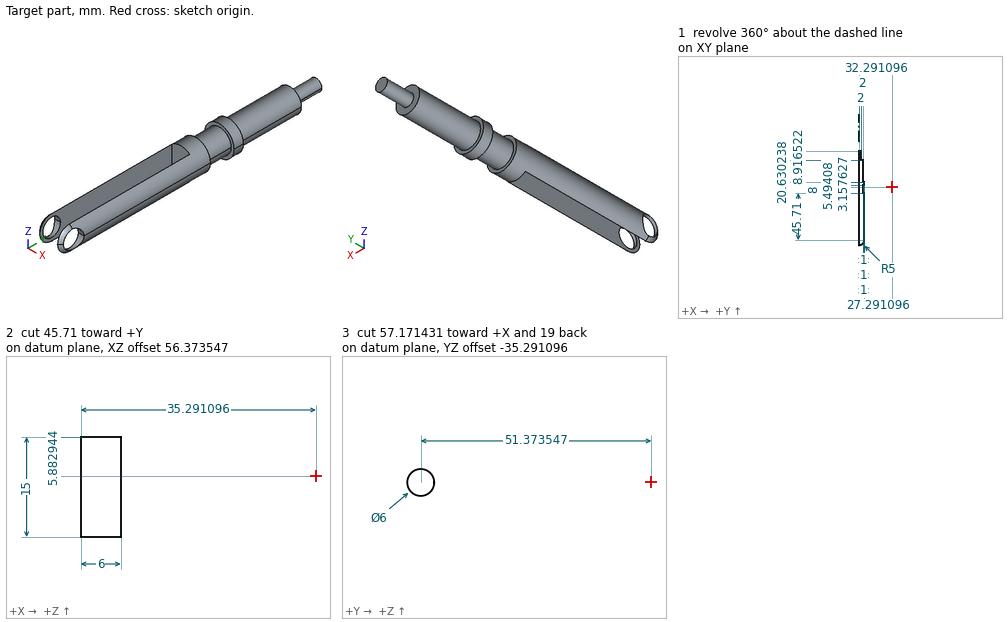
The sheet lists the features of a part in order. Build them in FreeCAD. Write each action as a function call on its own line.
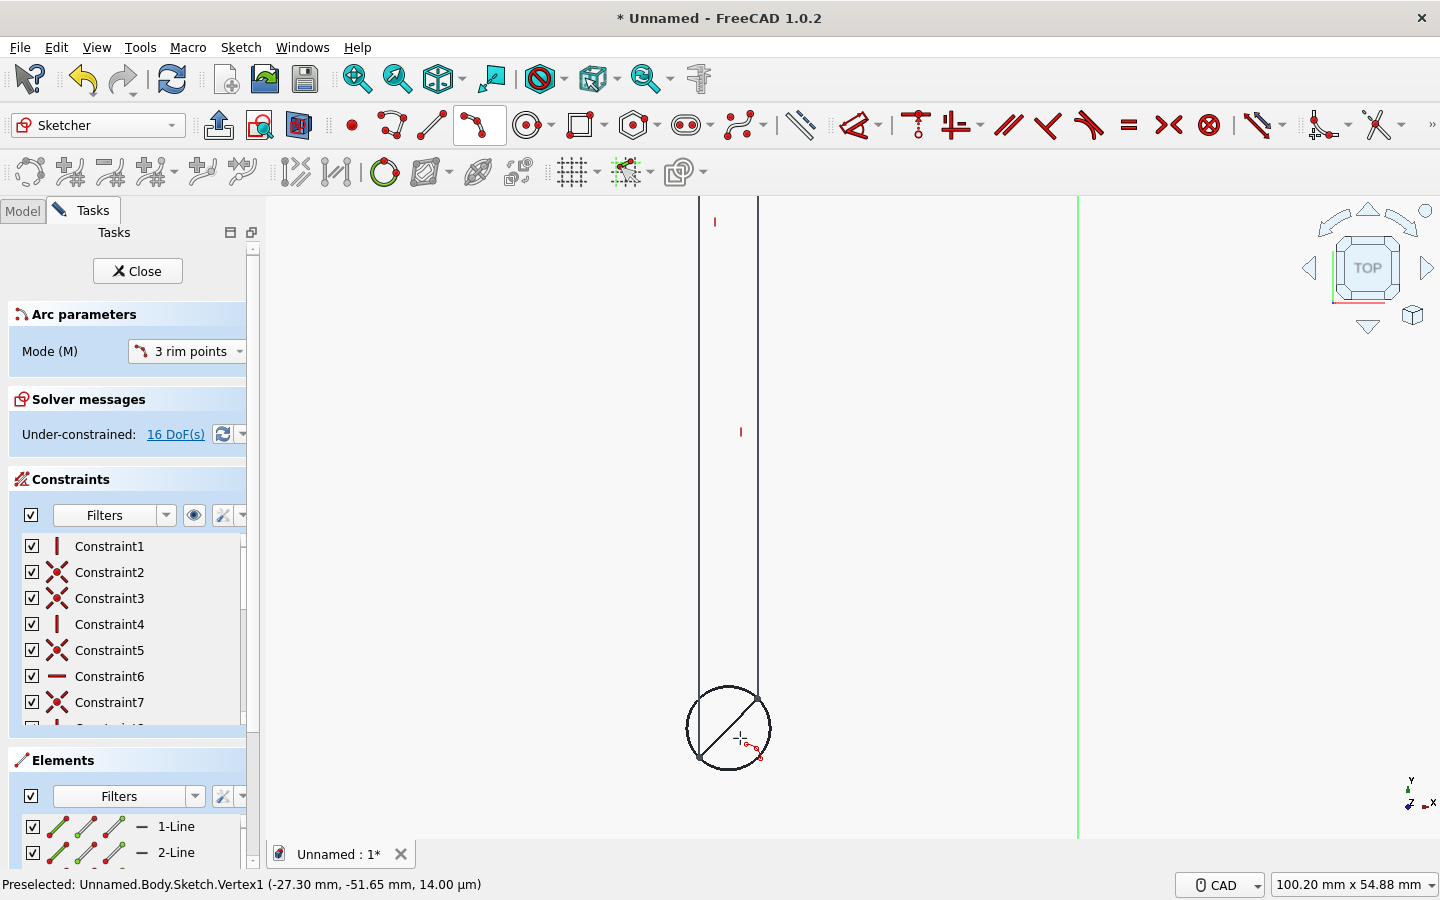
click(741, 737)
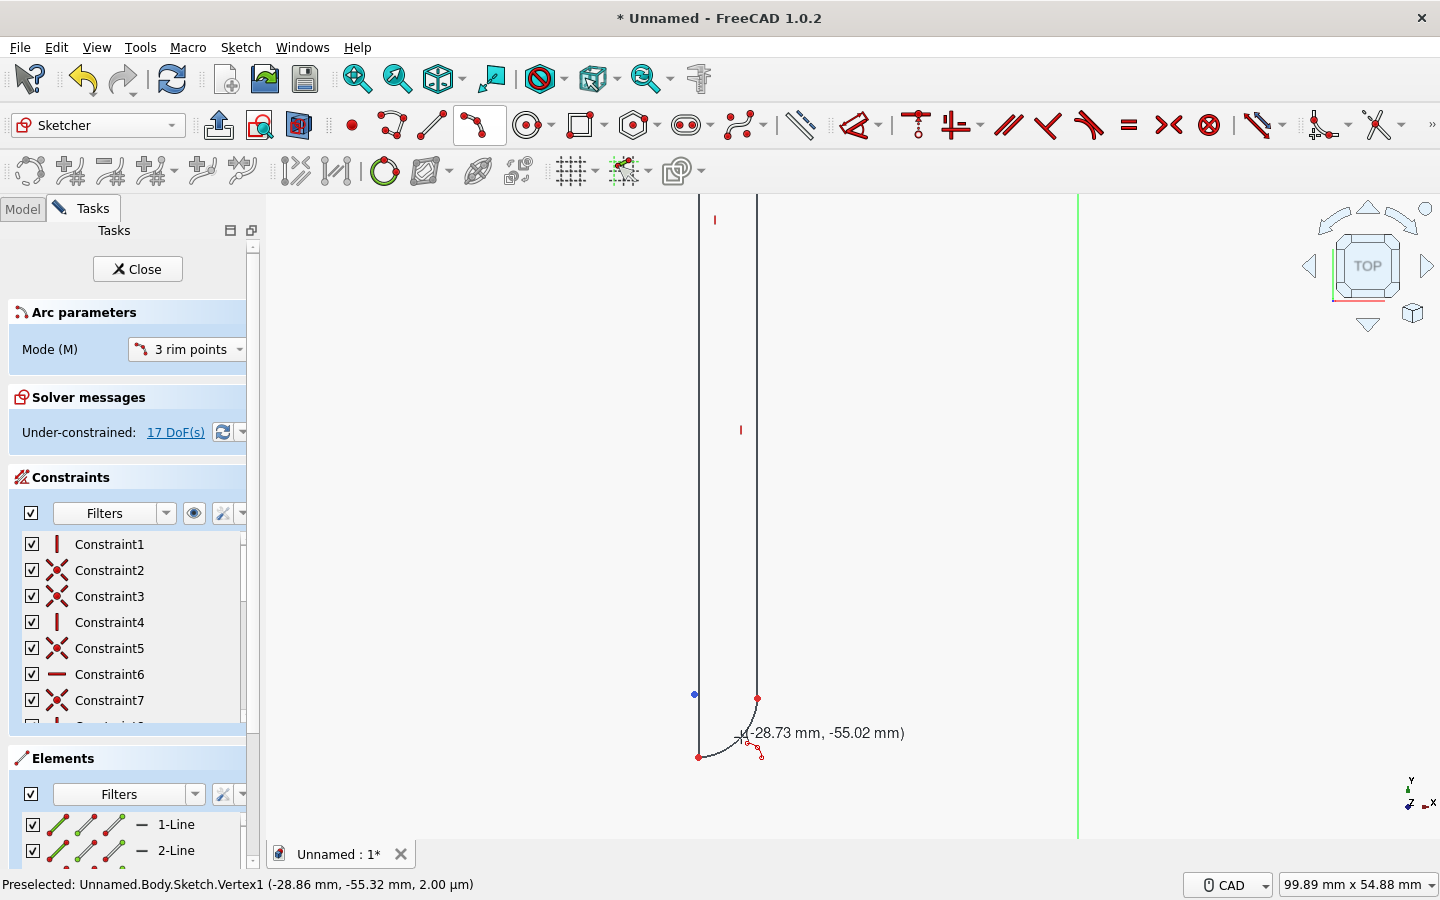
click(432, 126)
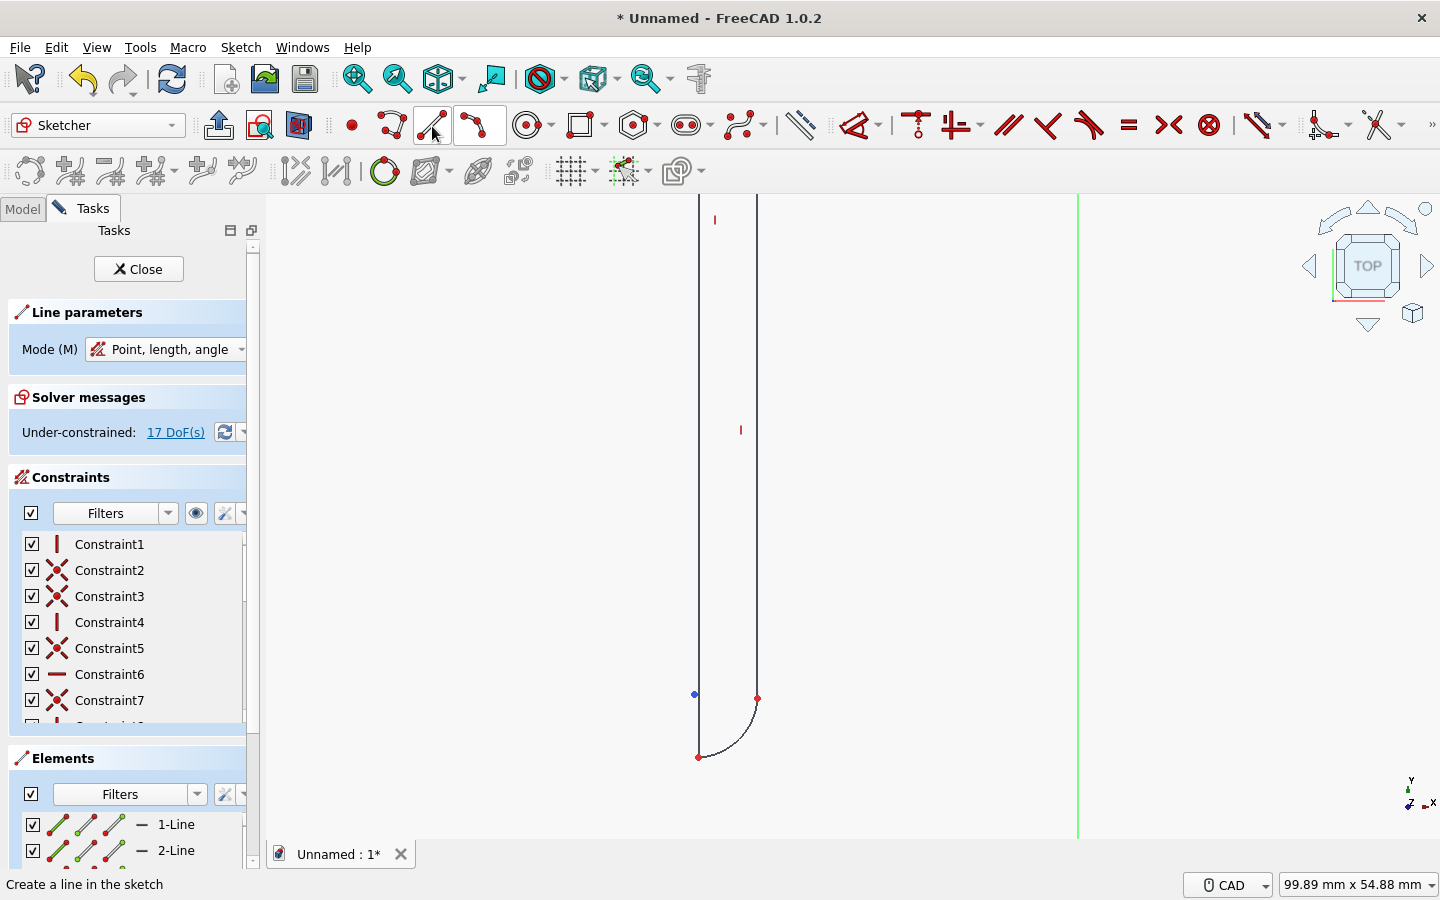
scroll(740, 738, down, 6)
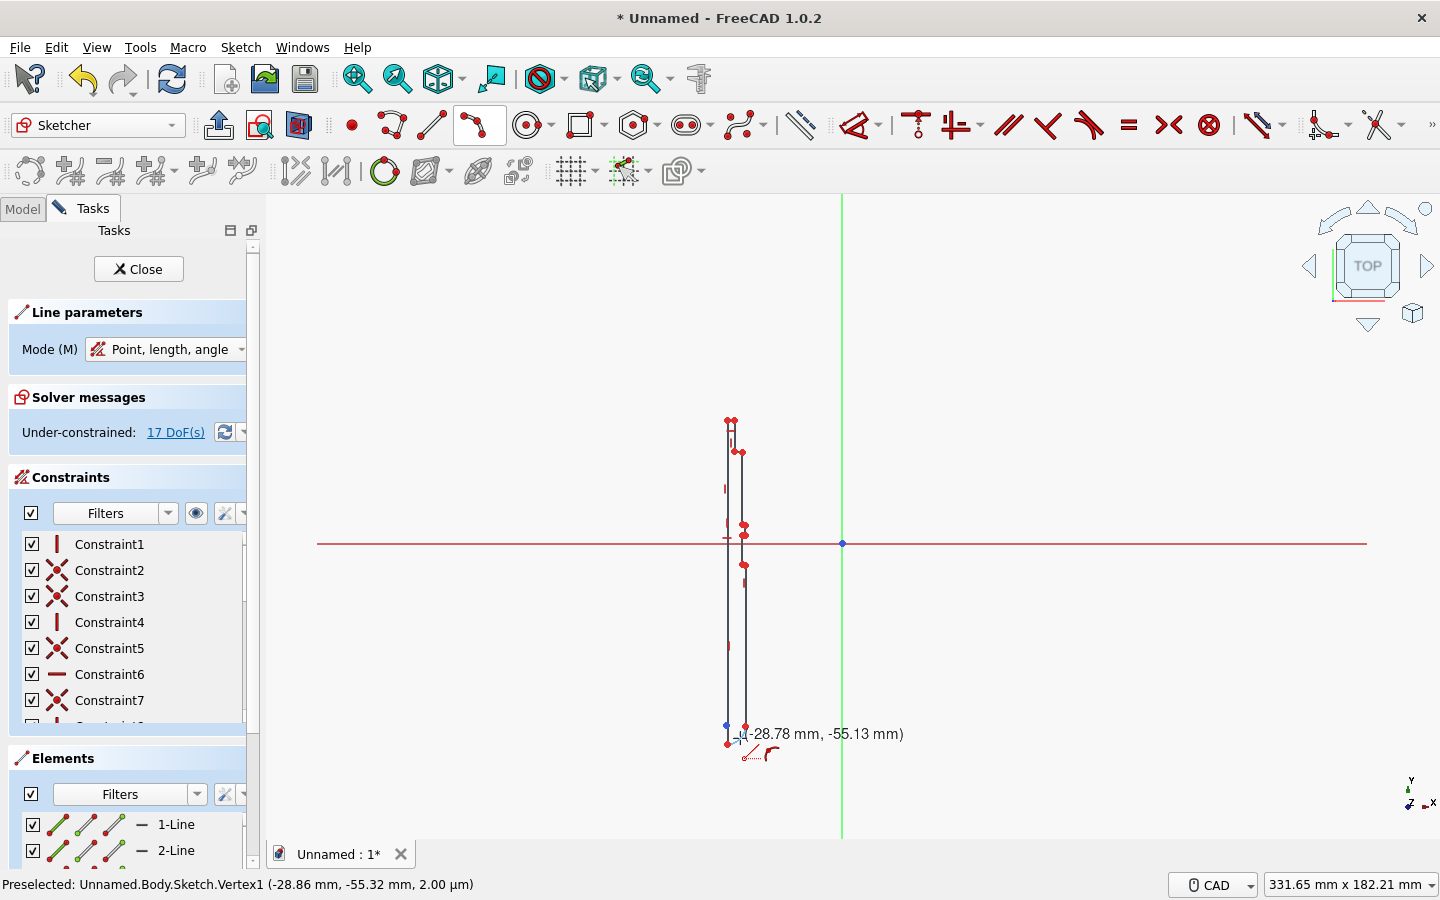
click(728, 387)
click(728, 290)
key(Escape)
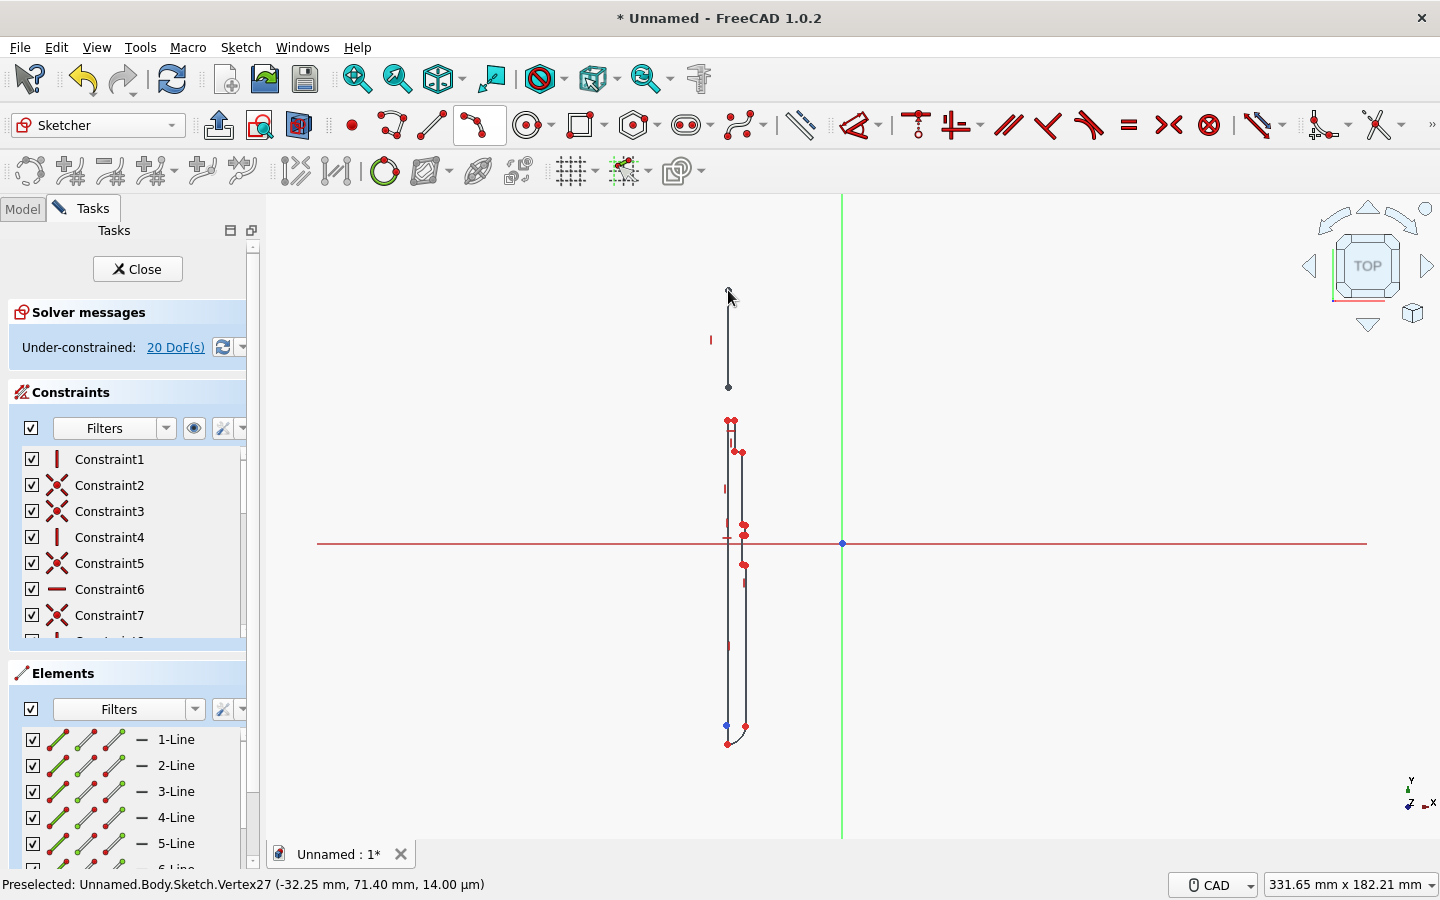
click(728, 359)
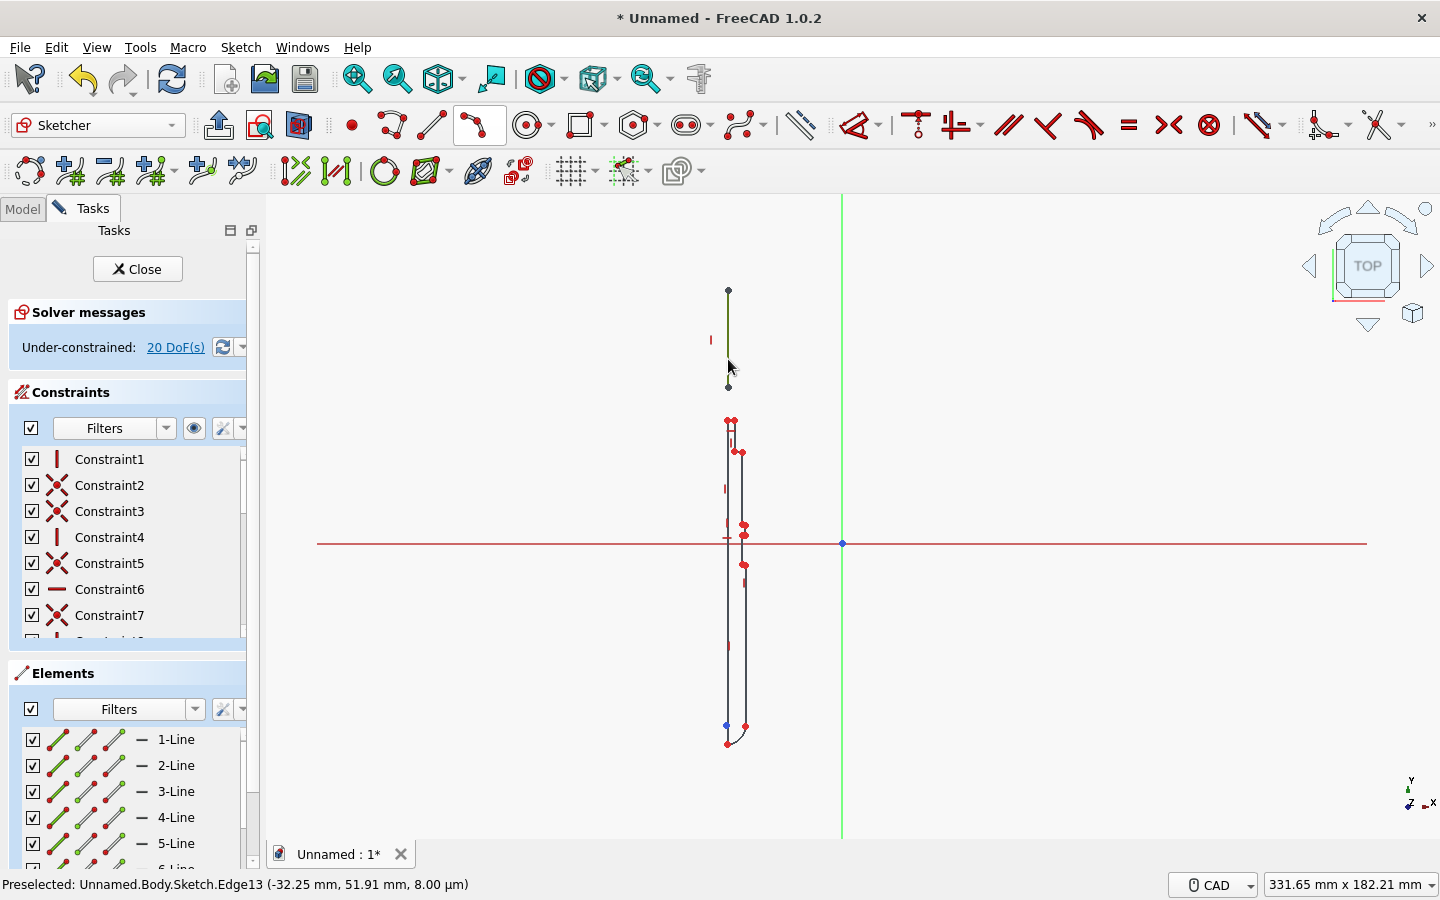
click(802, 126)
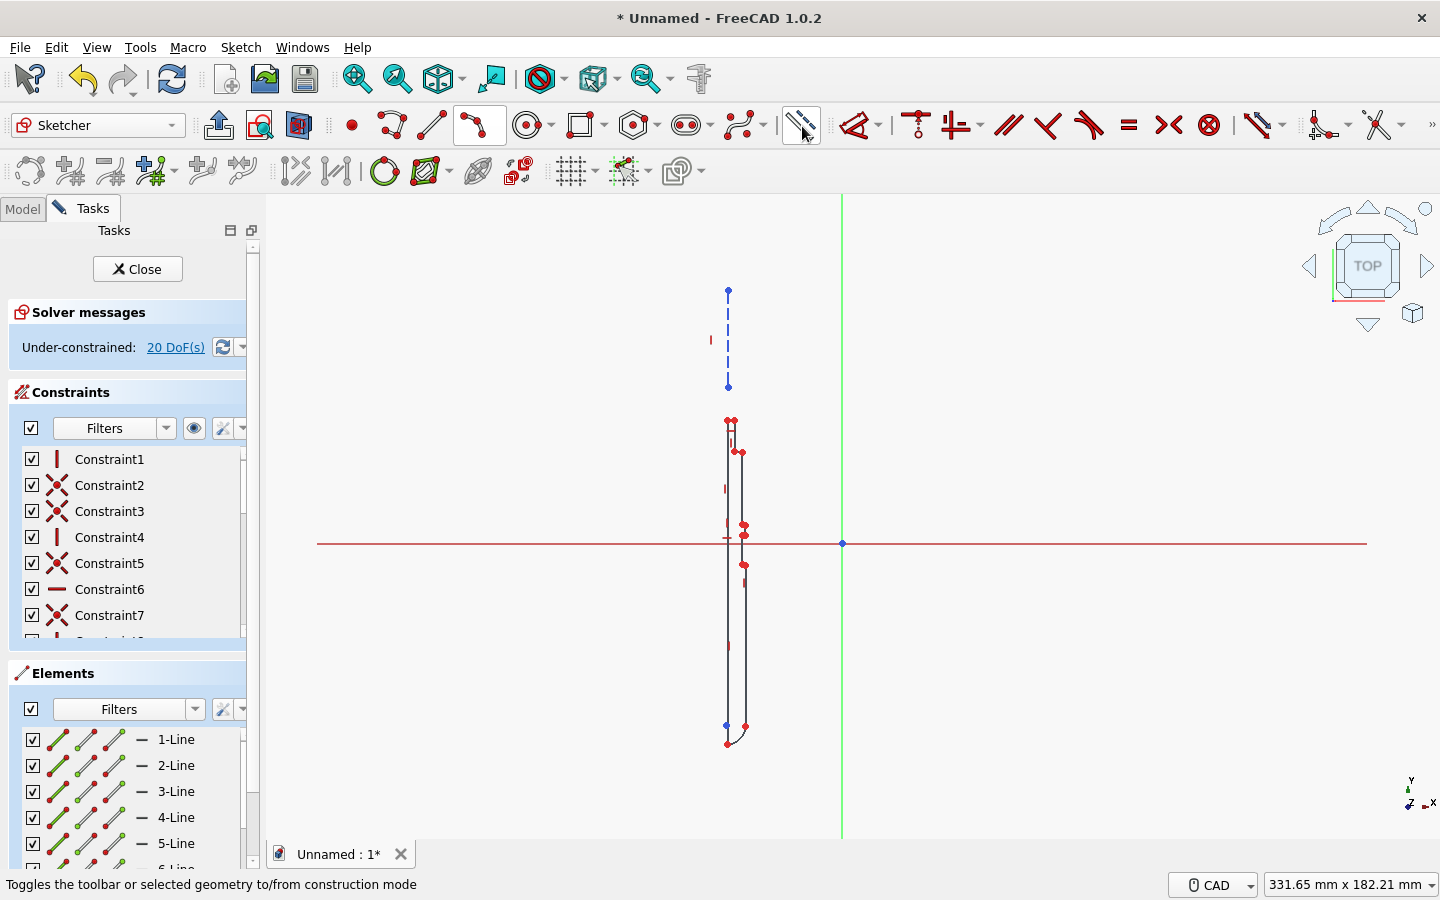
click(746, 678)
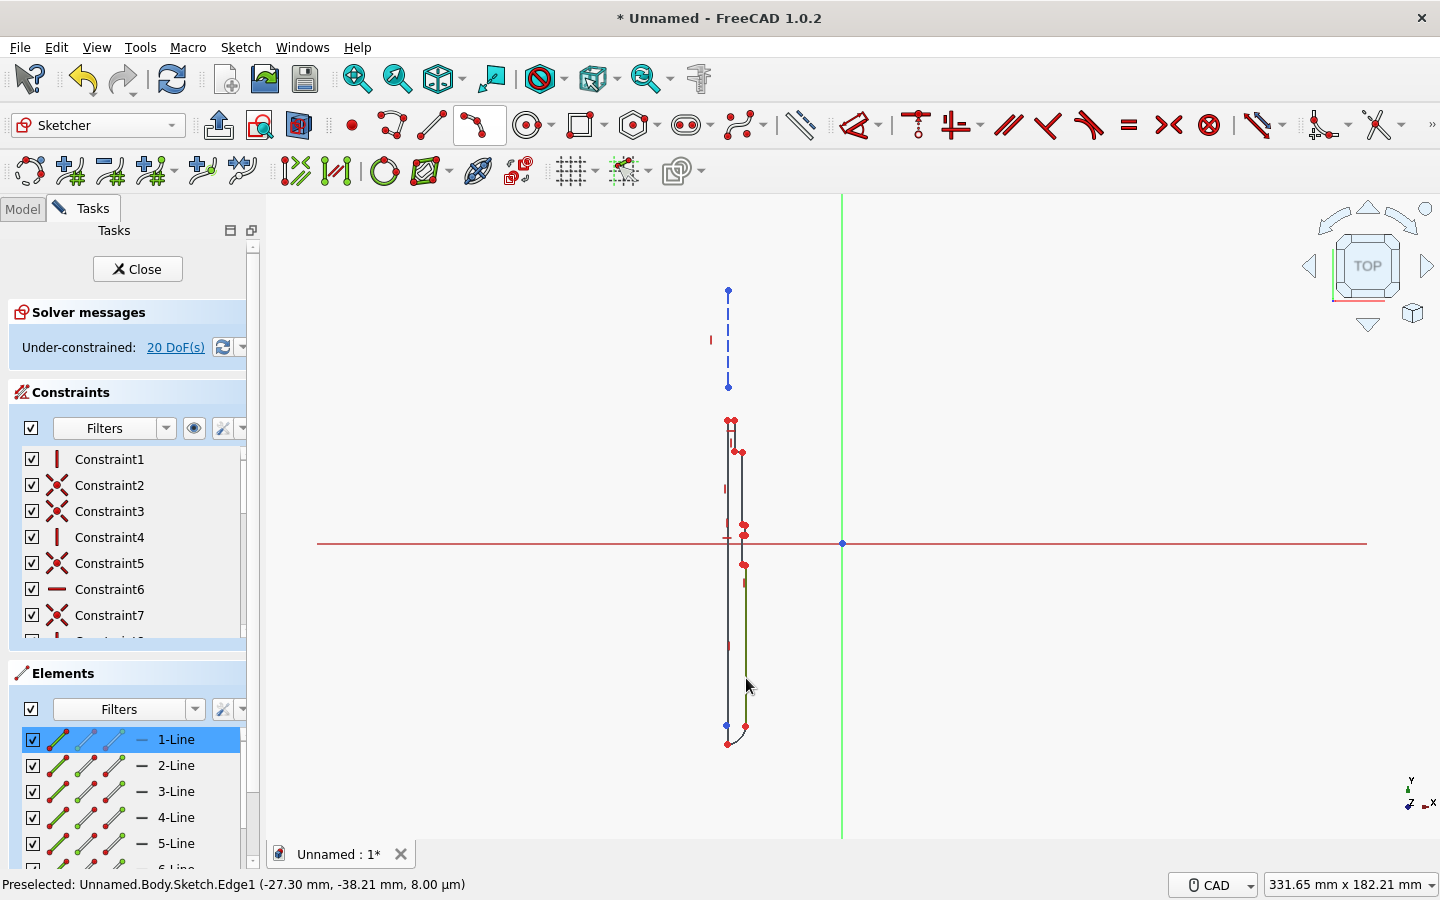
click(740, 739)